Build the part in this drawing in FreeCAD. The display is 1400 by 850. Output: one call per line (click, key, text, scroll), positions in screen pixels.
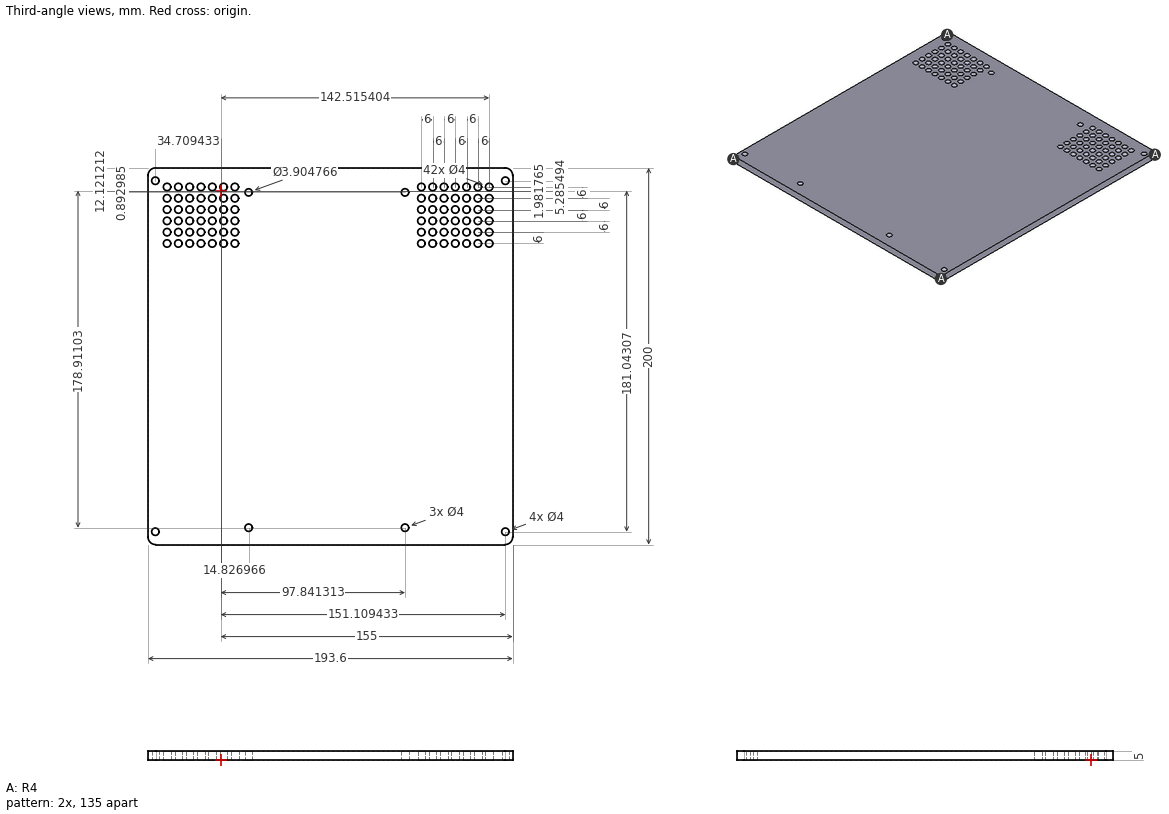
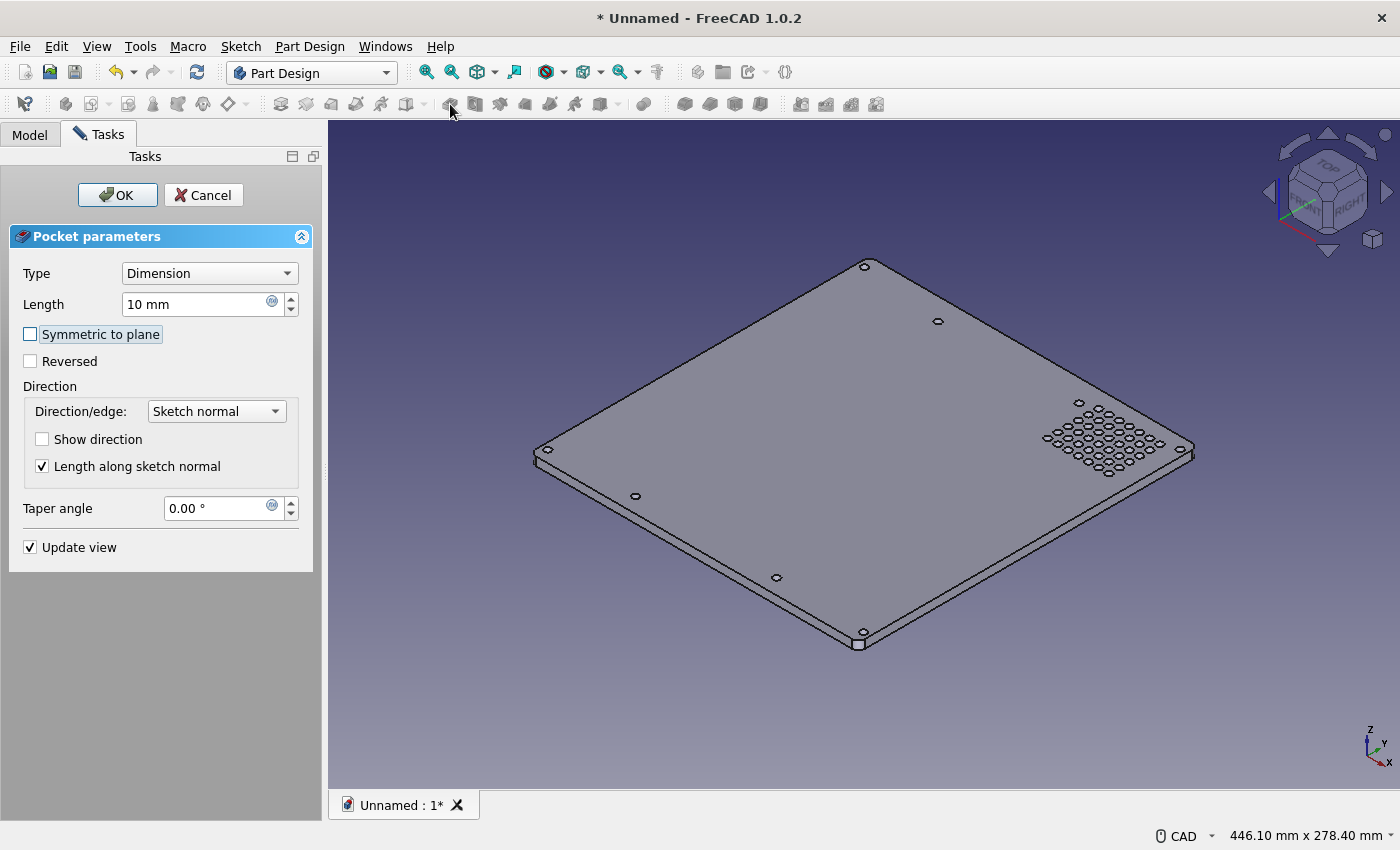
click(118, 195)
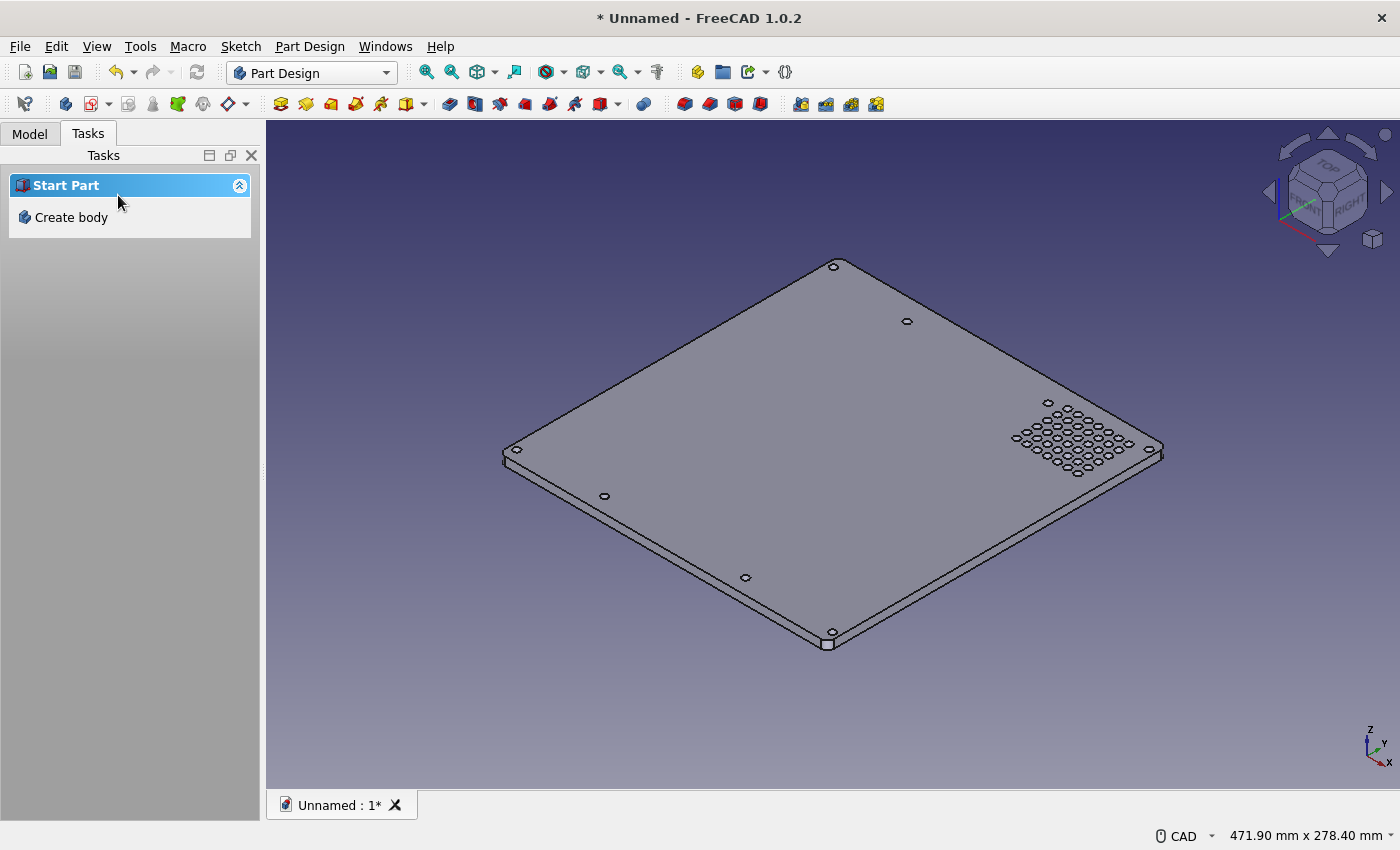
click(30, 134)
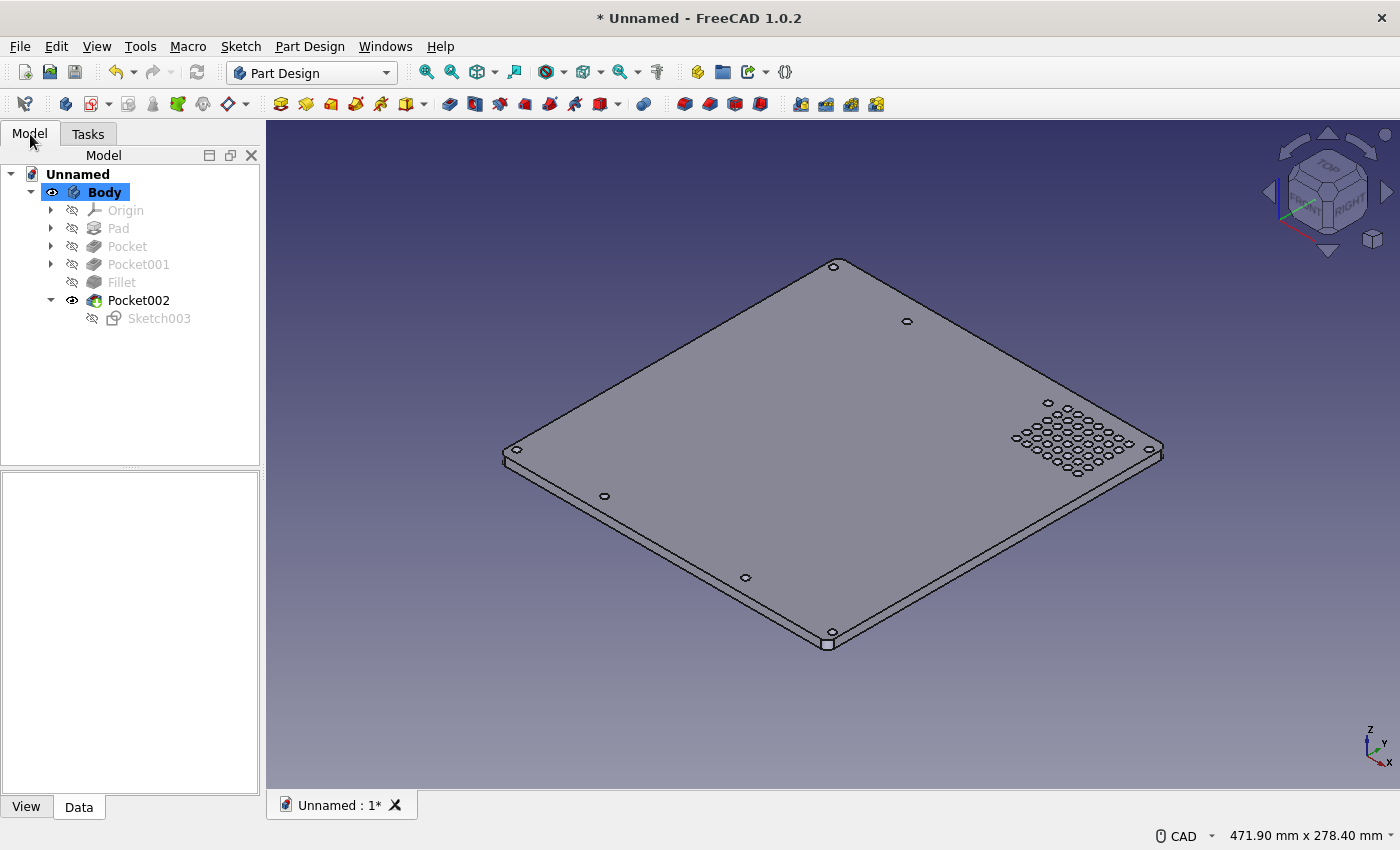
click(117, 300)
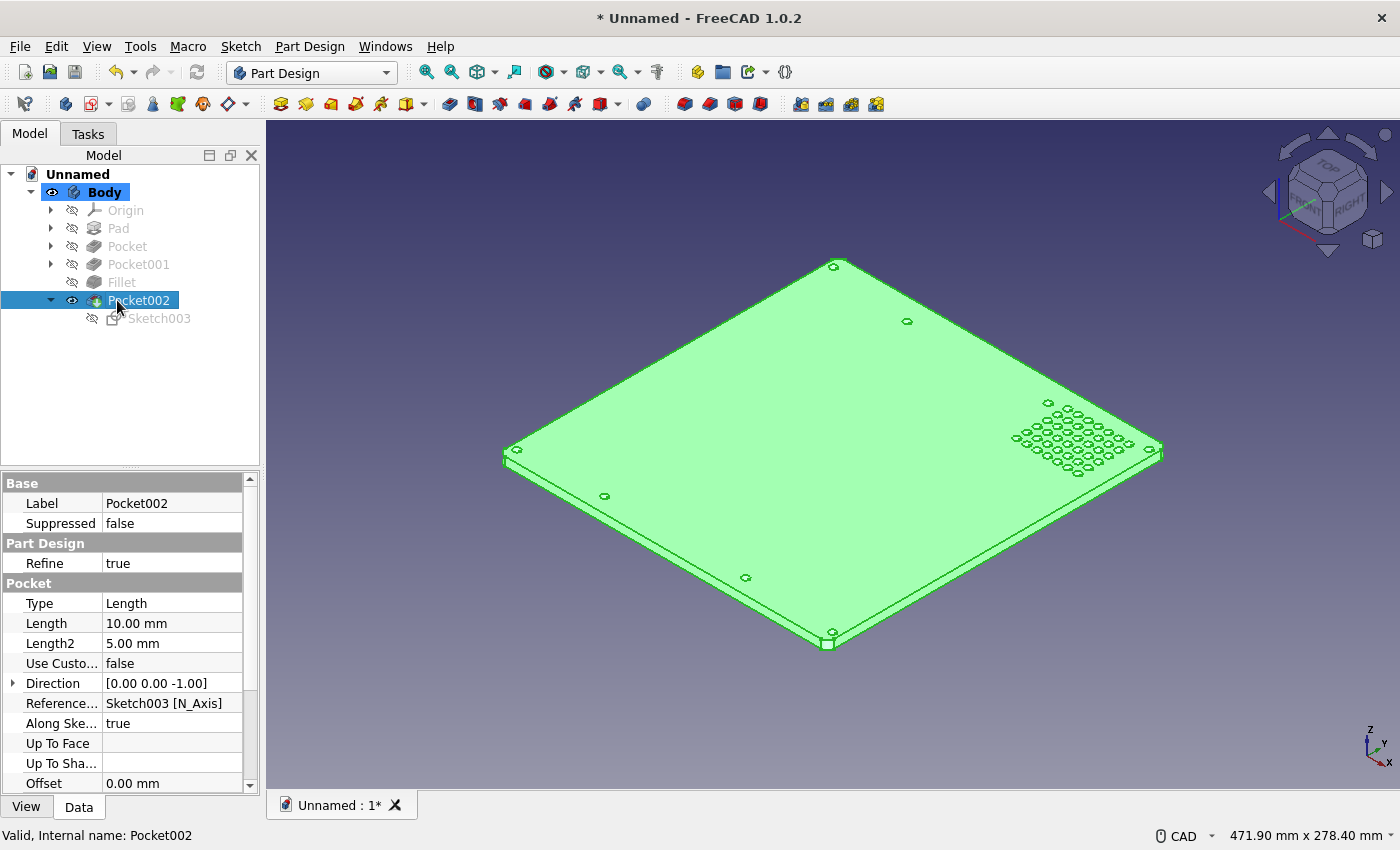
click(826, 104)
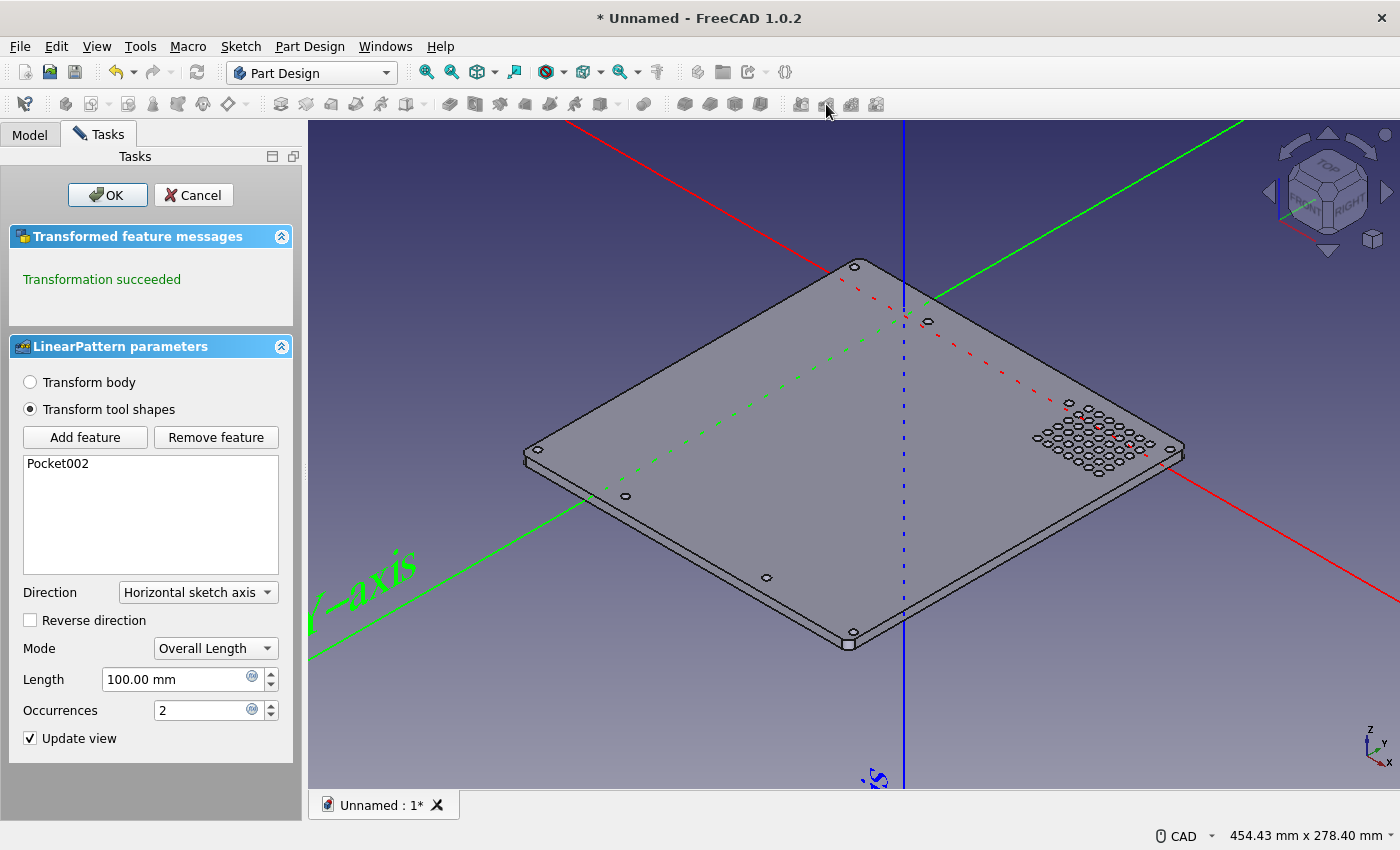
click(199, 592)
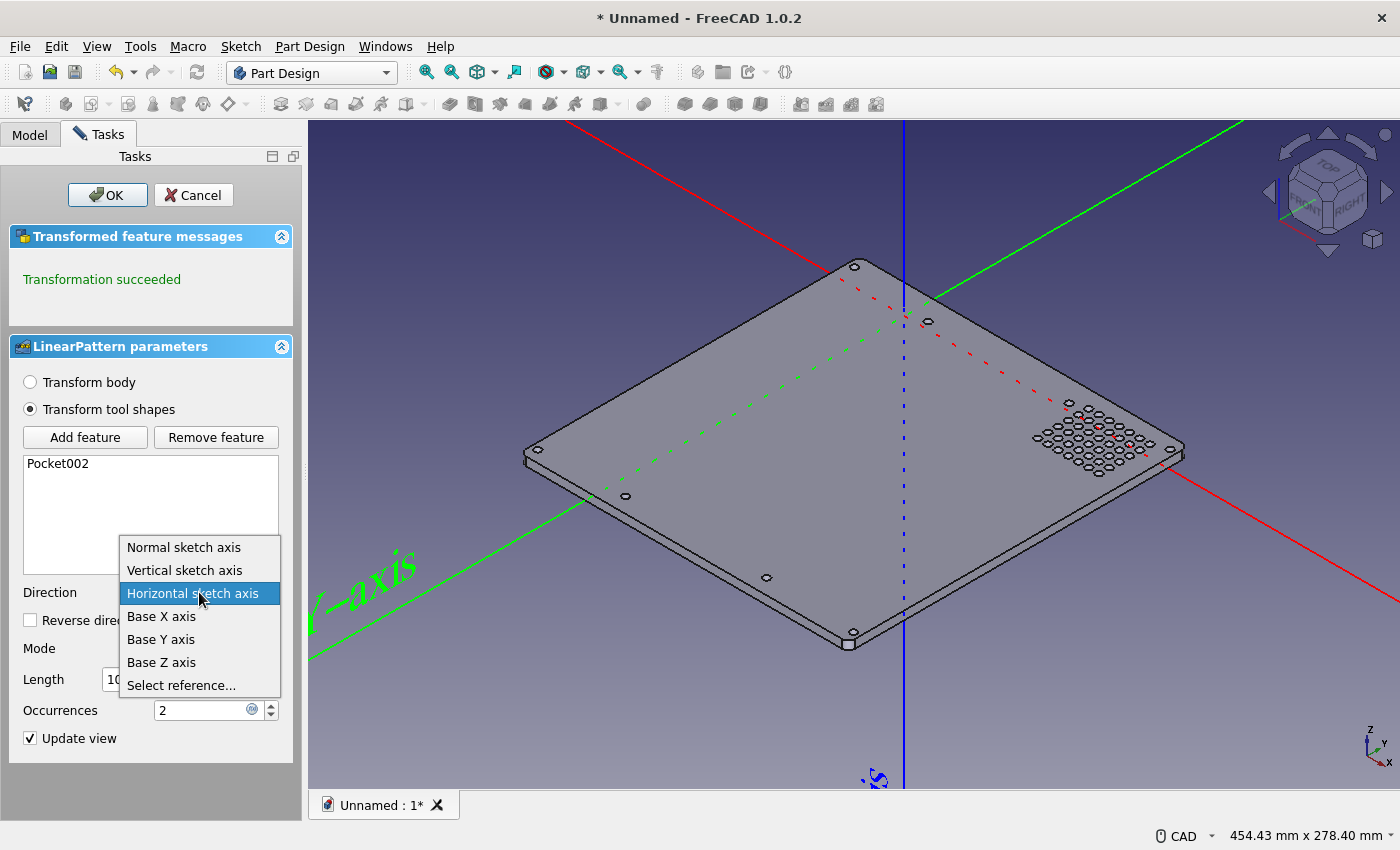
click(198, 616)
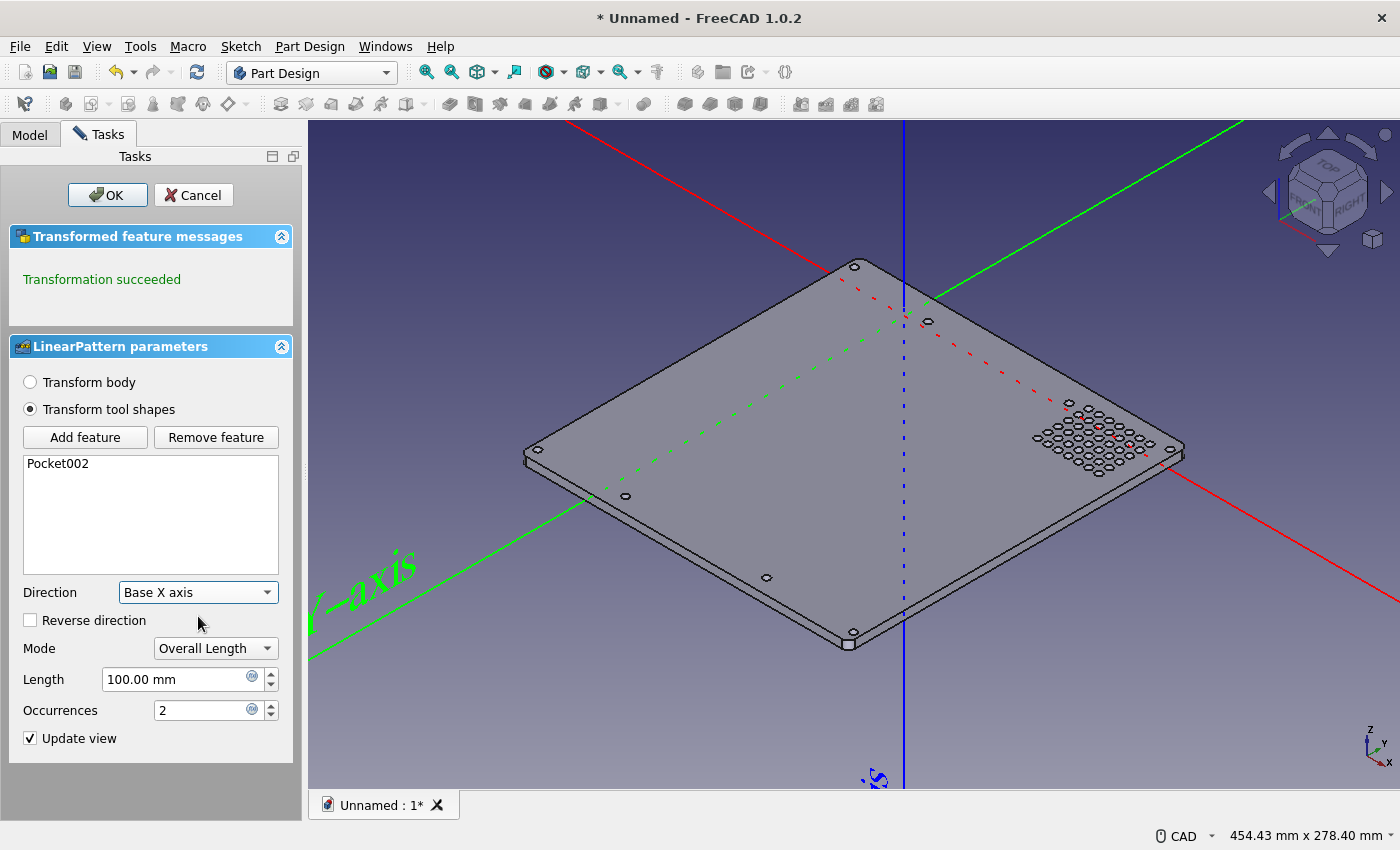
click(216, 648)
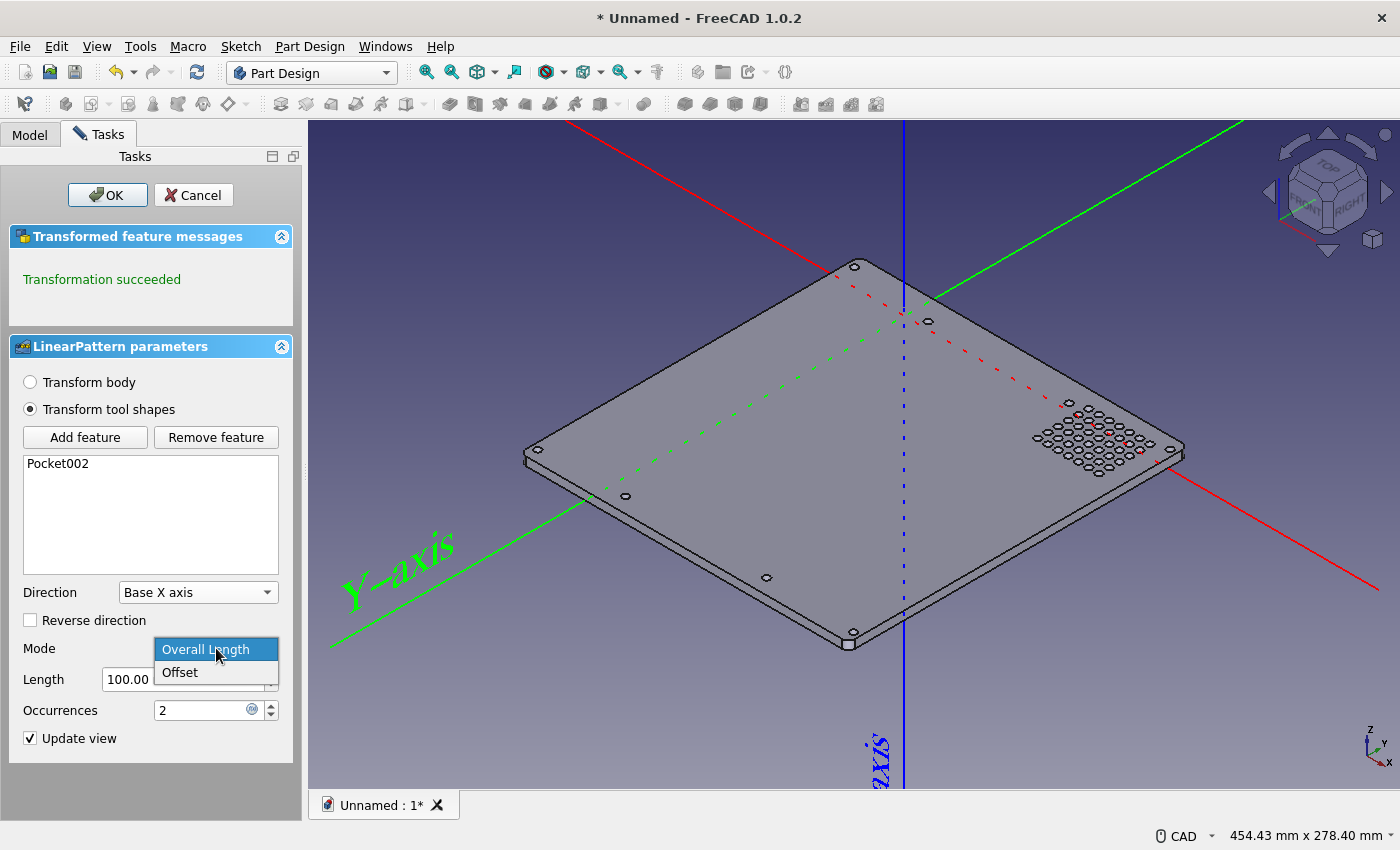
click(214, 672)